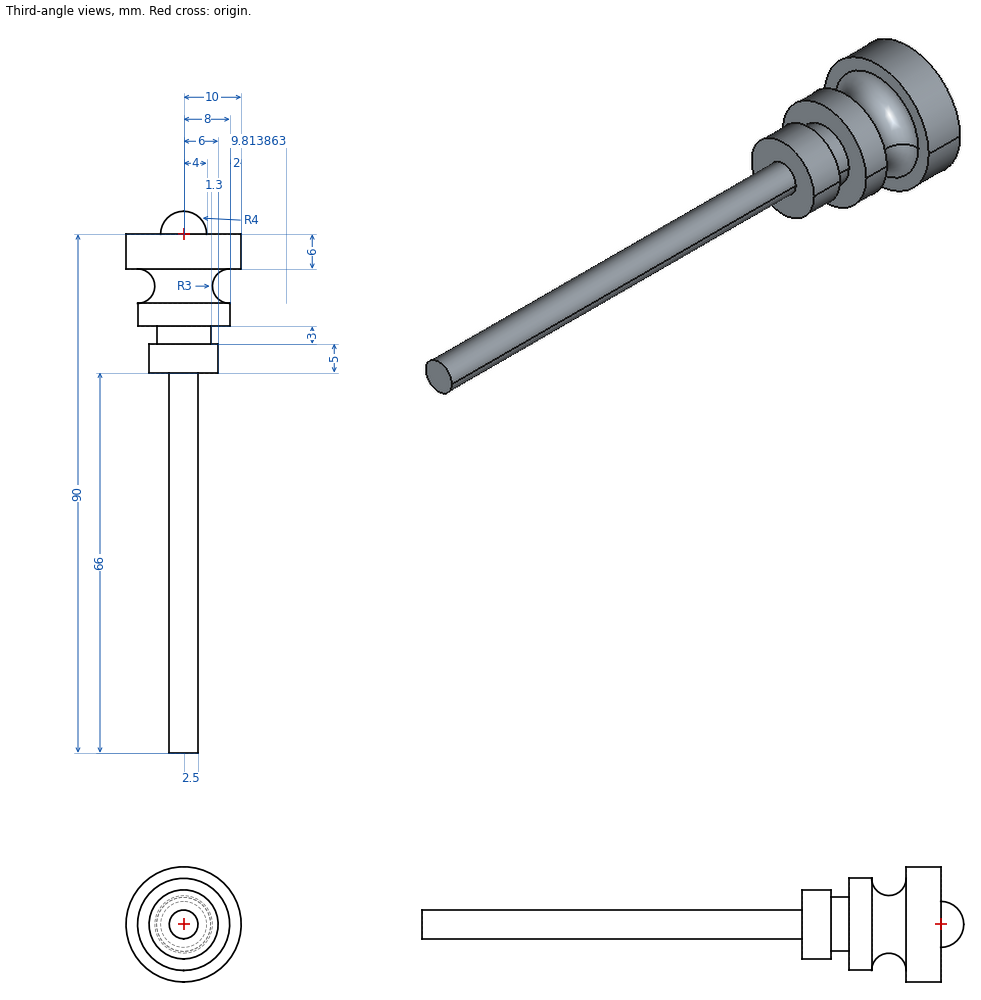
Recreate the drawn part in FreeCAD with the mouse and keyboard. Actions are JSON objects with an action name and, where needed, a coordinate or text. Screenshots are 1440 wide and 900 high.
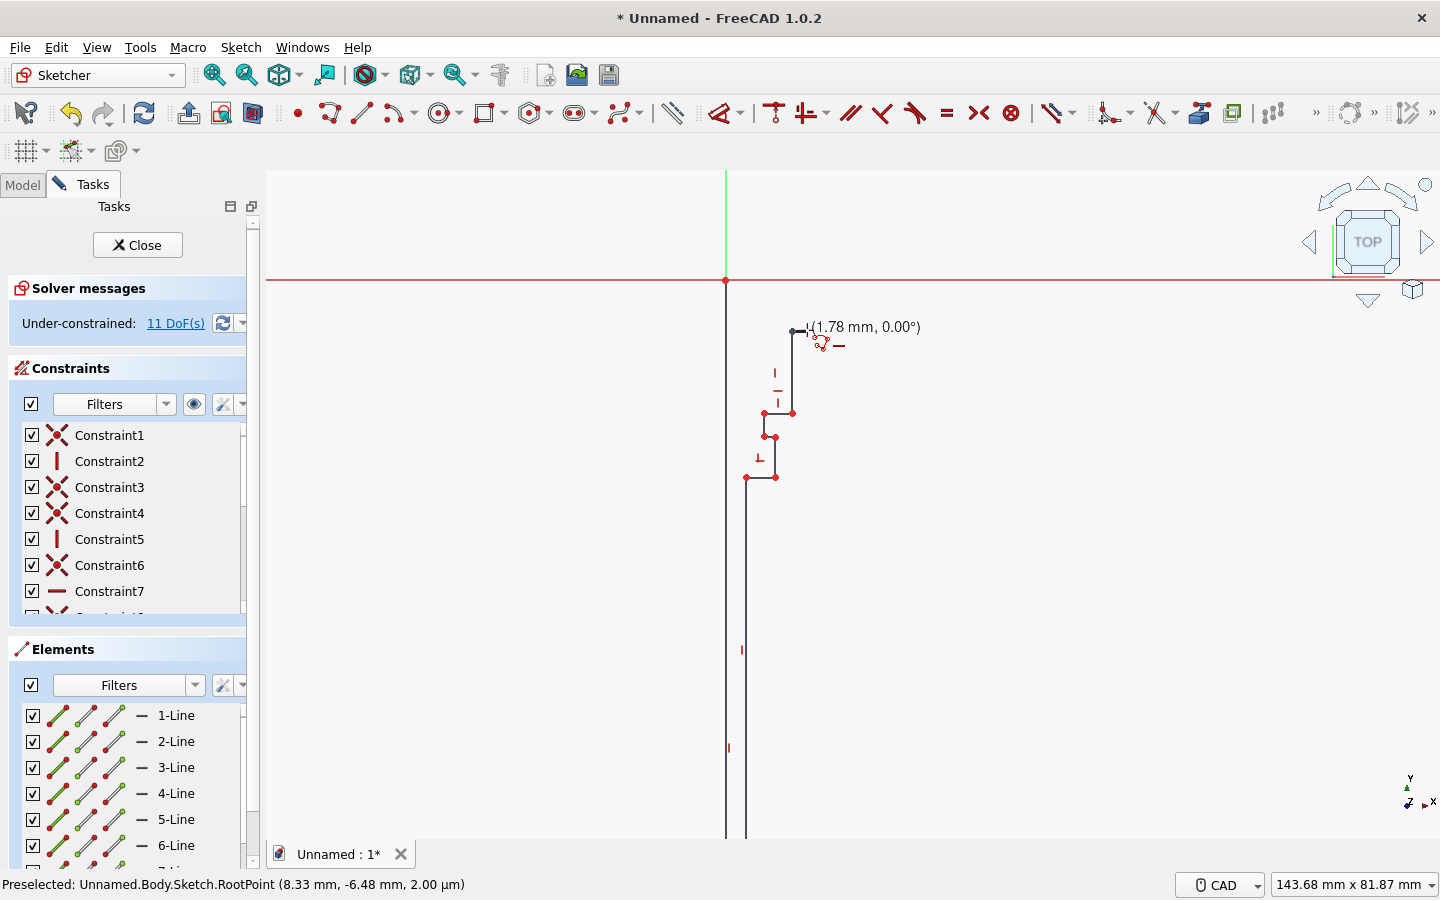
{"action": "left_click", "coordinate": [808, 330]}
{"action": "left_click", "coordinate": [808, 289]}
{"action": "left_click", "coordinate": [726, 280]}
{"action": "key", "text": "Escape"}
{"action": "key", "text": "Escape"}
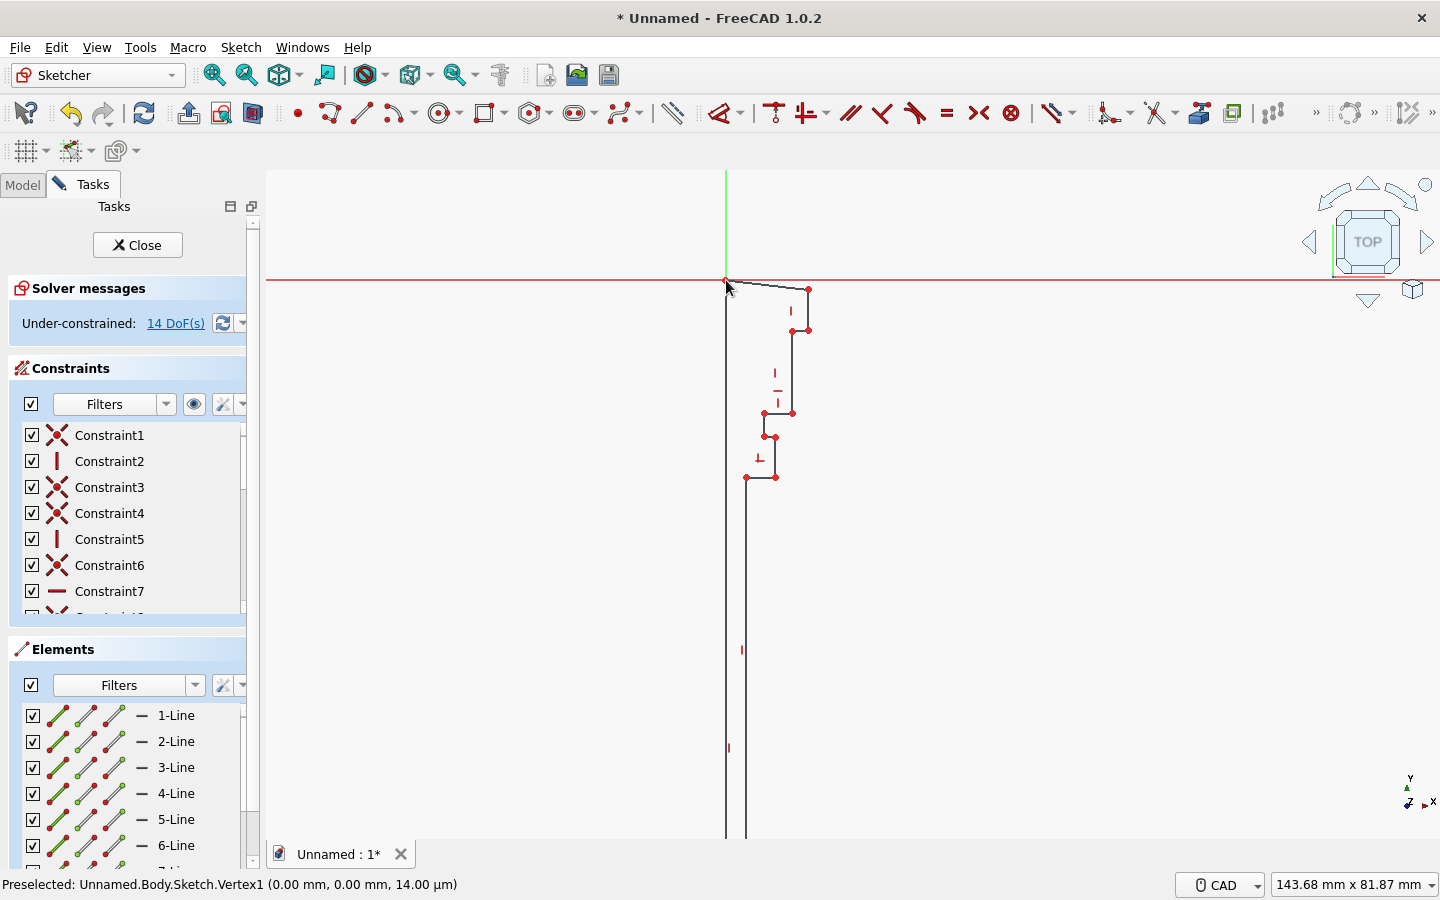
{"action": "scroll", "coordinate": [806, 330], "scroll_direction": "down", "scroll_amount": 3}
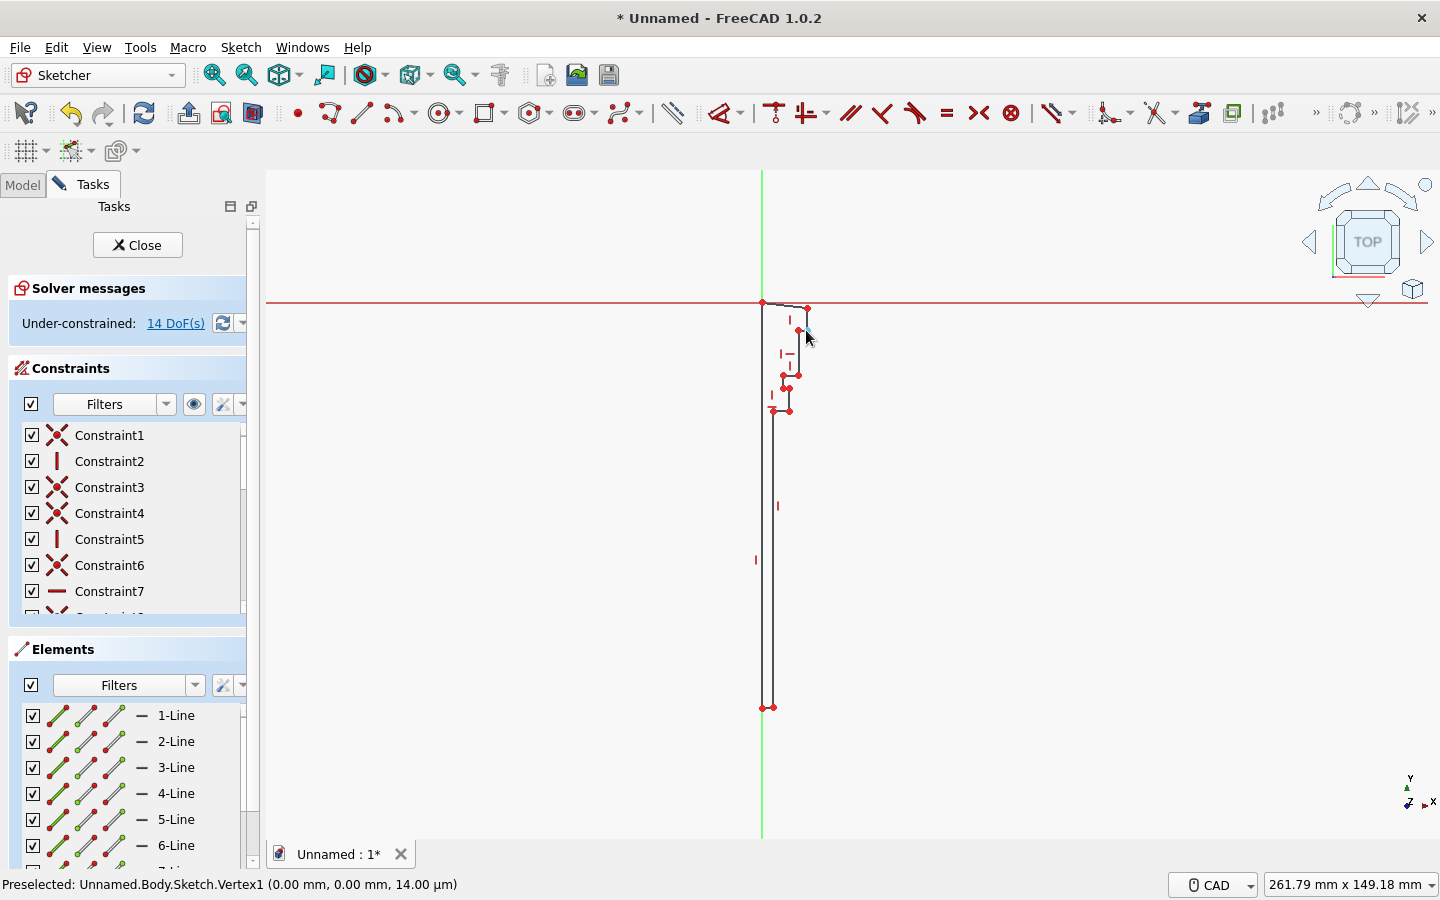
{"action": "scroll", "coordinate": [768, 708], "scroll_direction": "up", "scroll_amount": 5}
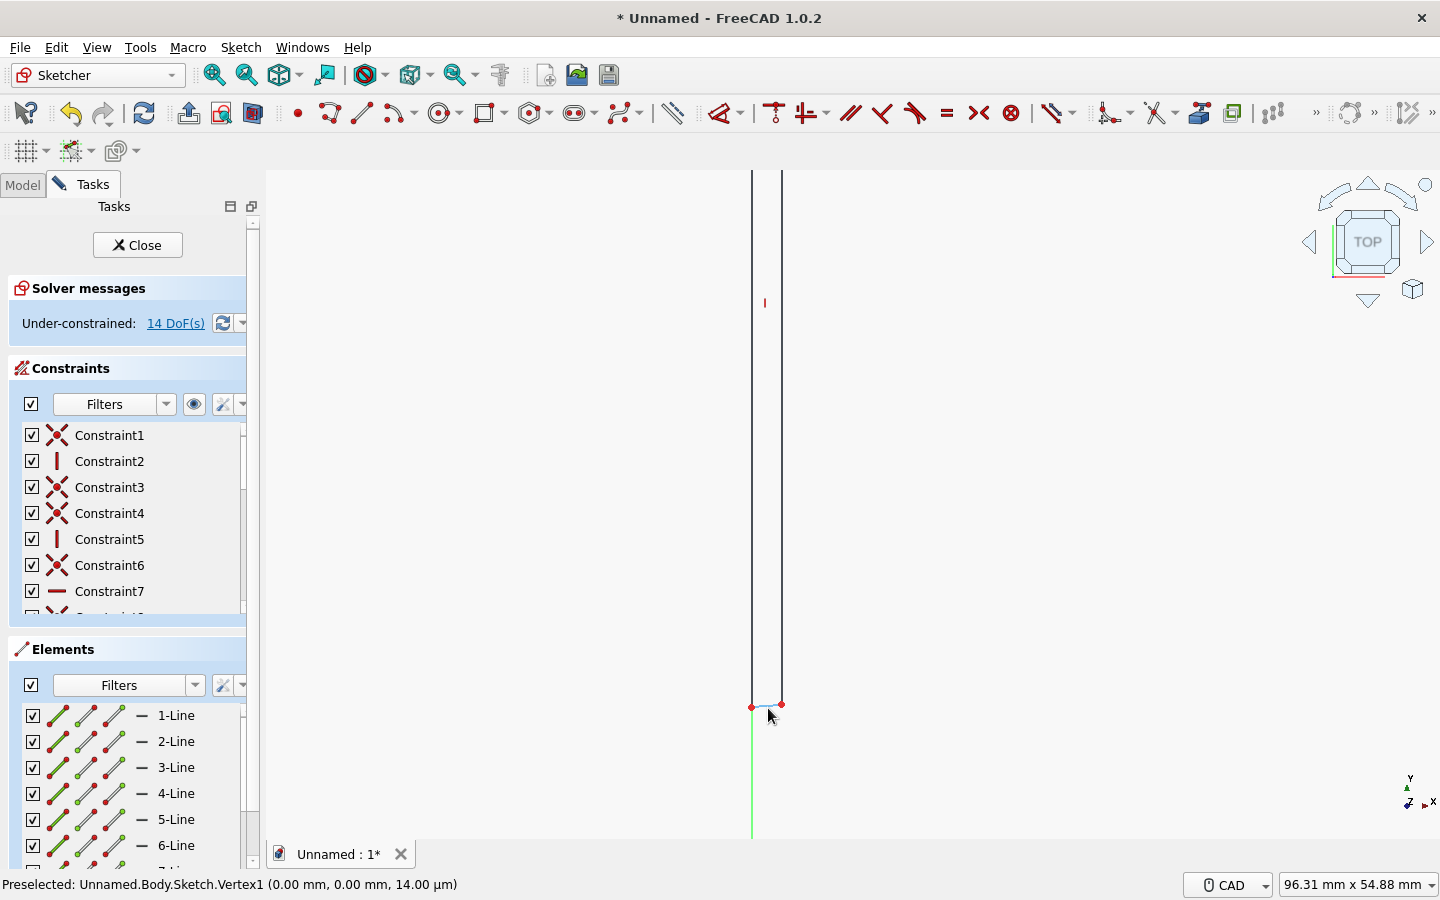
{"action": "left_click", "coordinate": [767, 706]}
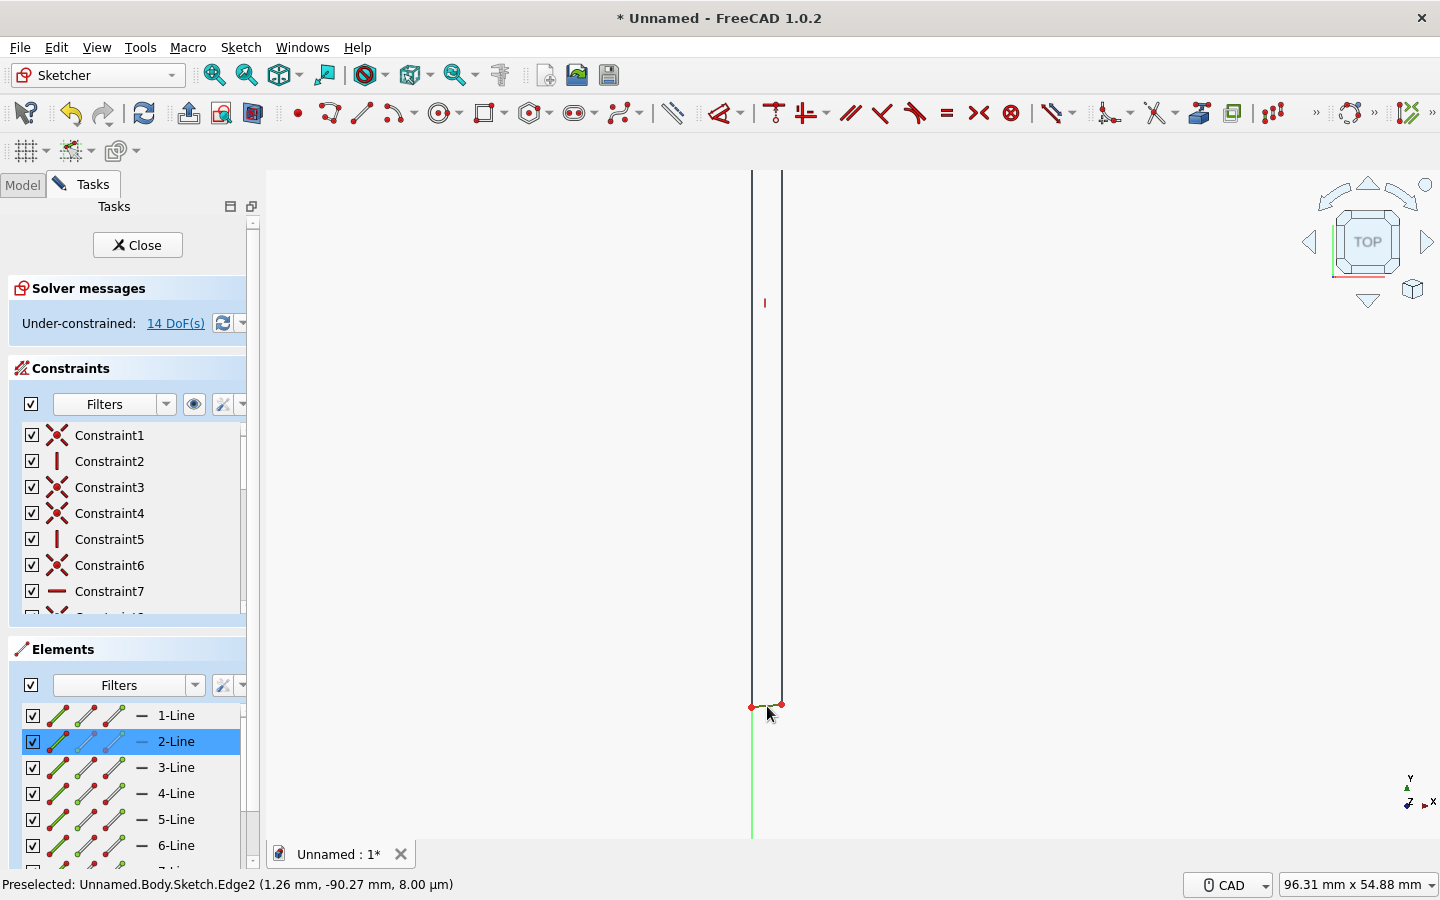
{"action": "key", "text": "h"}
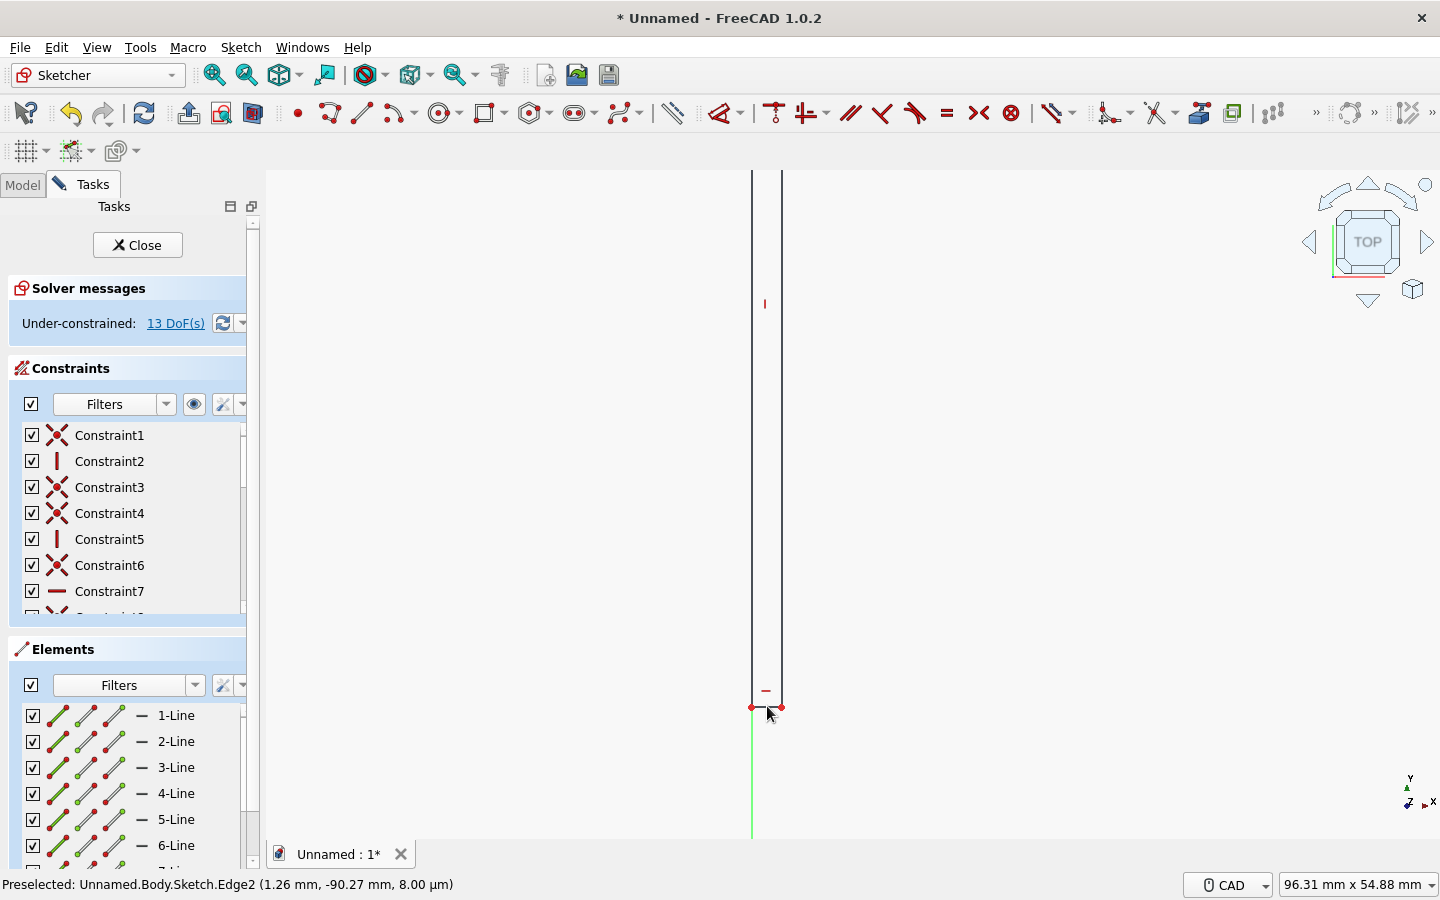
{"action": "scroll", "coordinate": [768, 708], "scroll_direction": "down", "scroll_amount": 5}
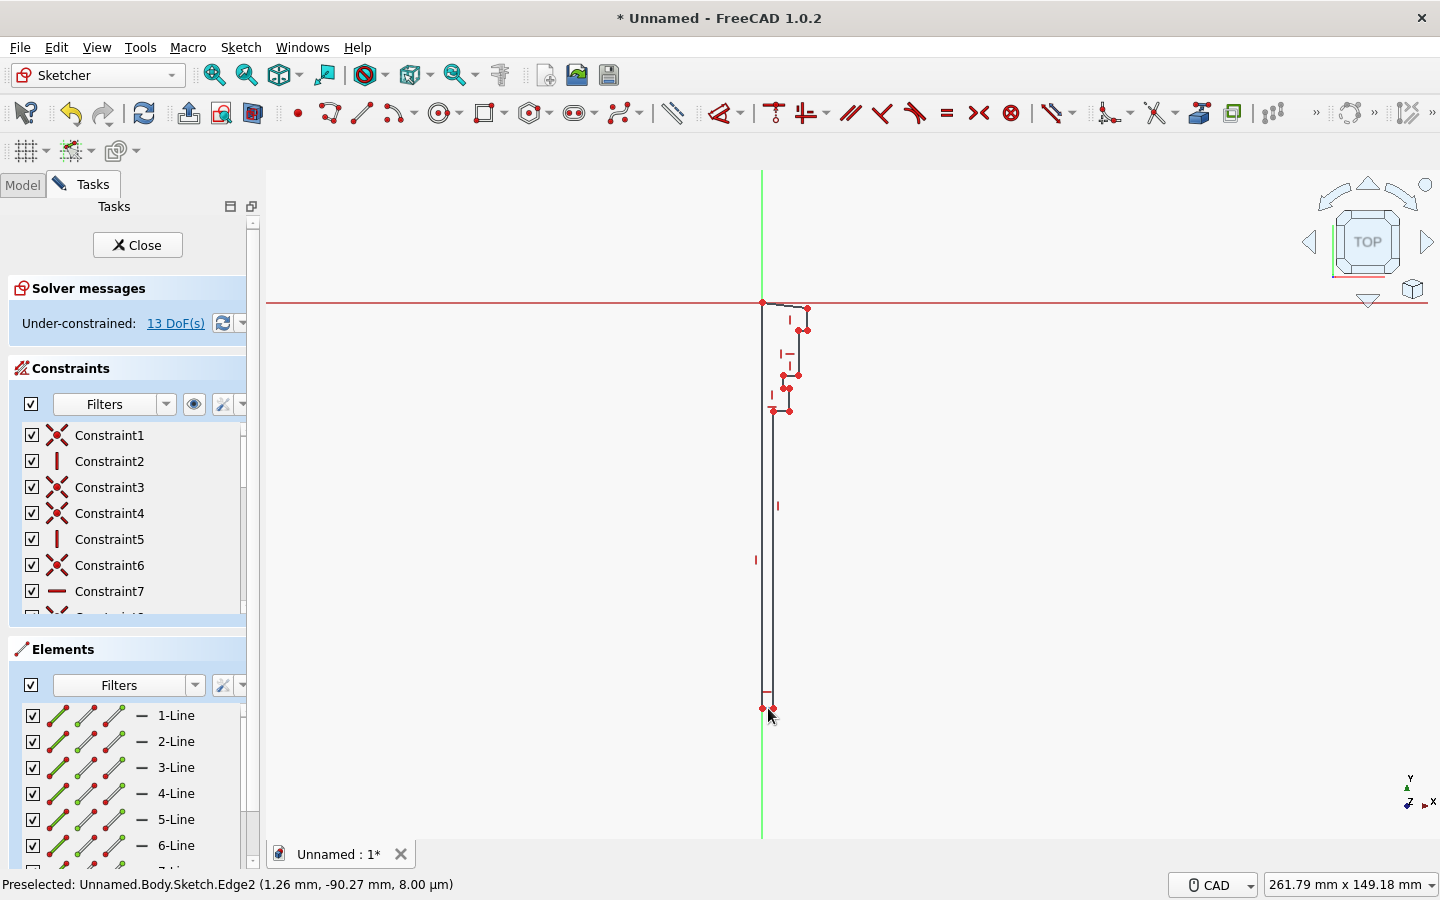
{"action": "scroll", "coordinate": [786, 389], "scroll_direction": "up", "scroll_amount": 8}